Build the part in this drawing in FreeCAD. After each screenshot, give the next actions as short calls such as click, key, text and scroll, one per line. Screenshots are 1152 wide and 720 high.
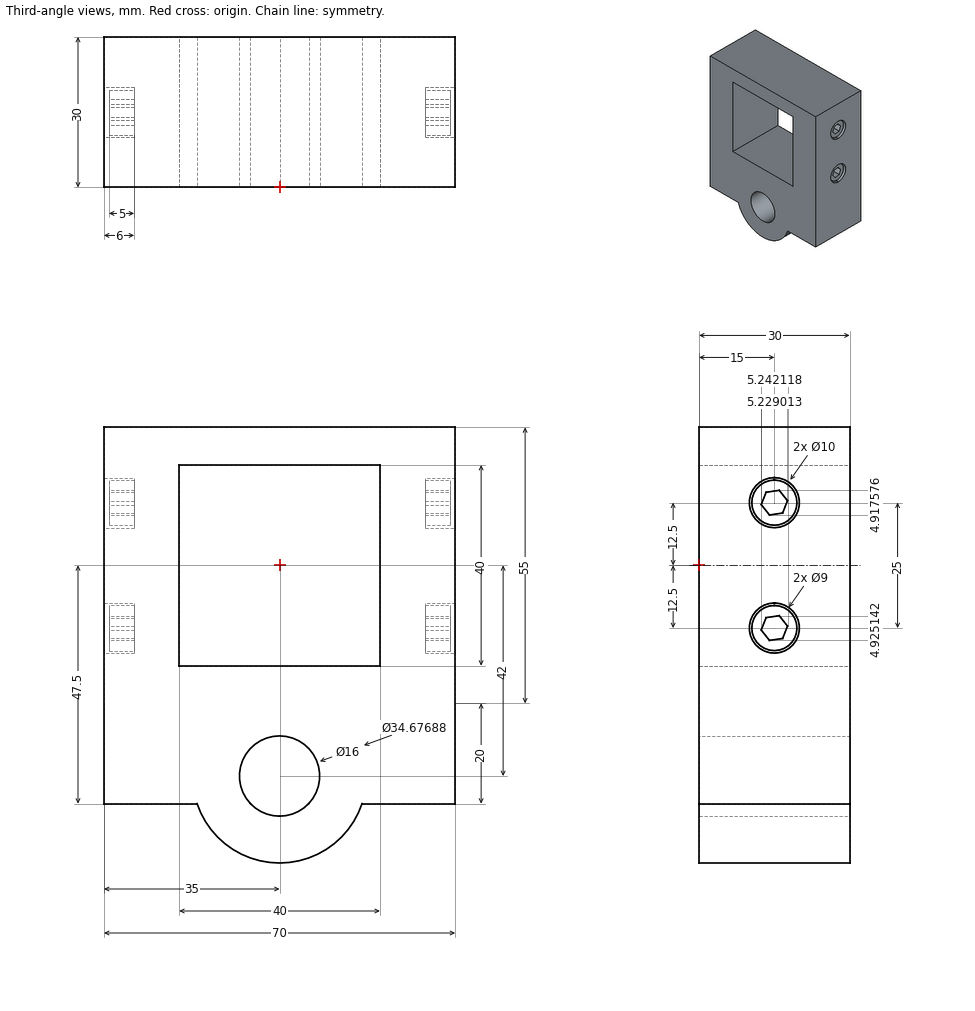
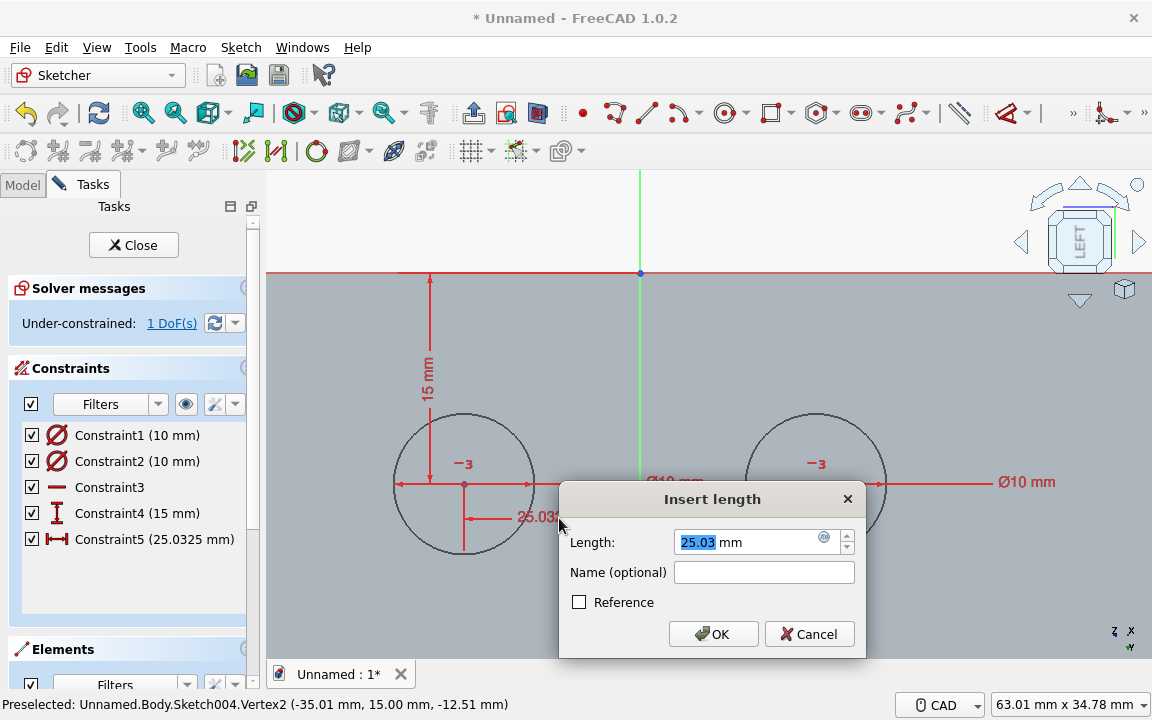
text(25)
key(Return)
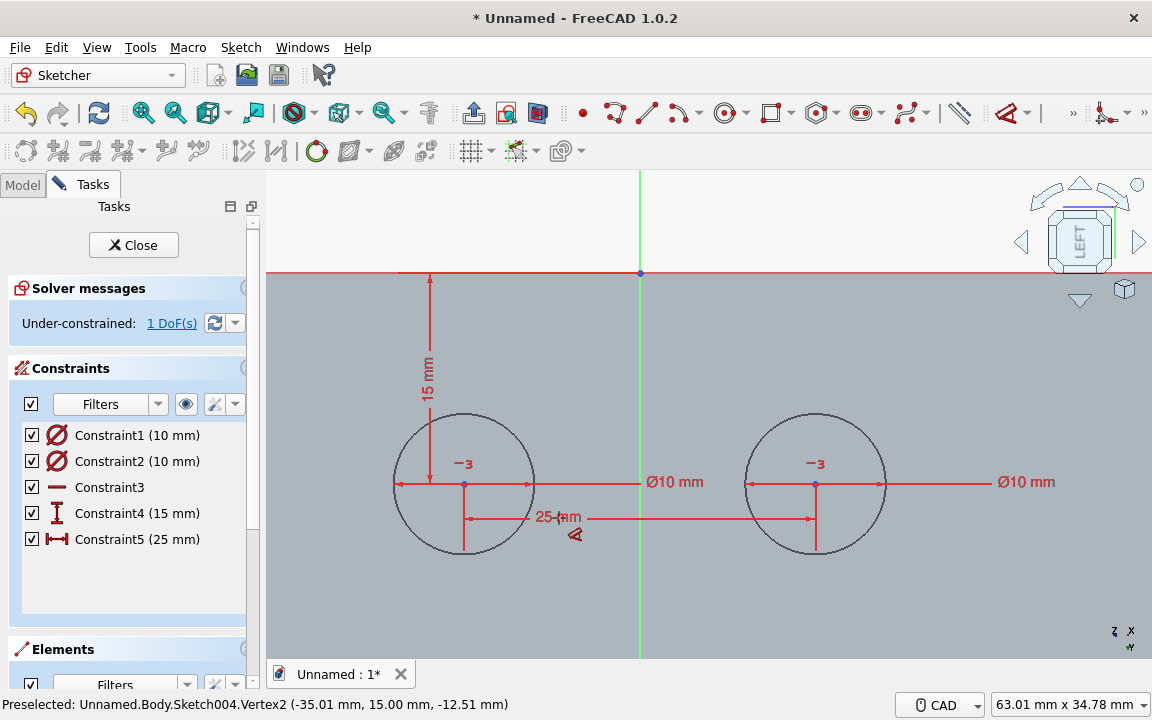
click(464, 484)
click(552, 239)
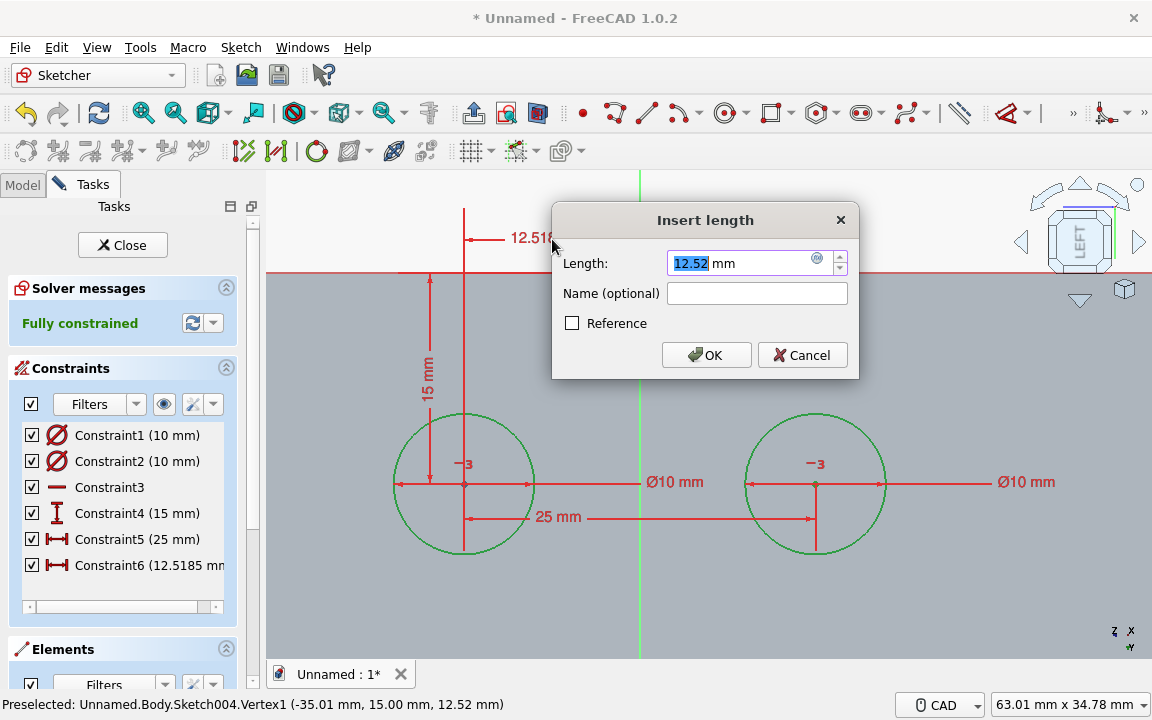
text(12.5)
key(Return)
key(Escape)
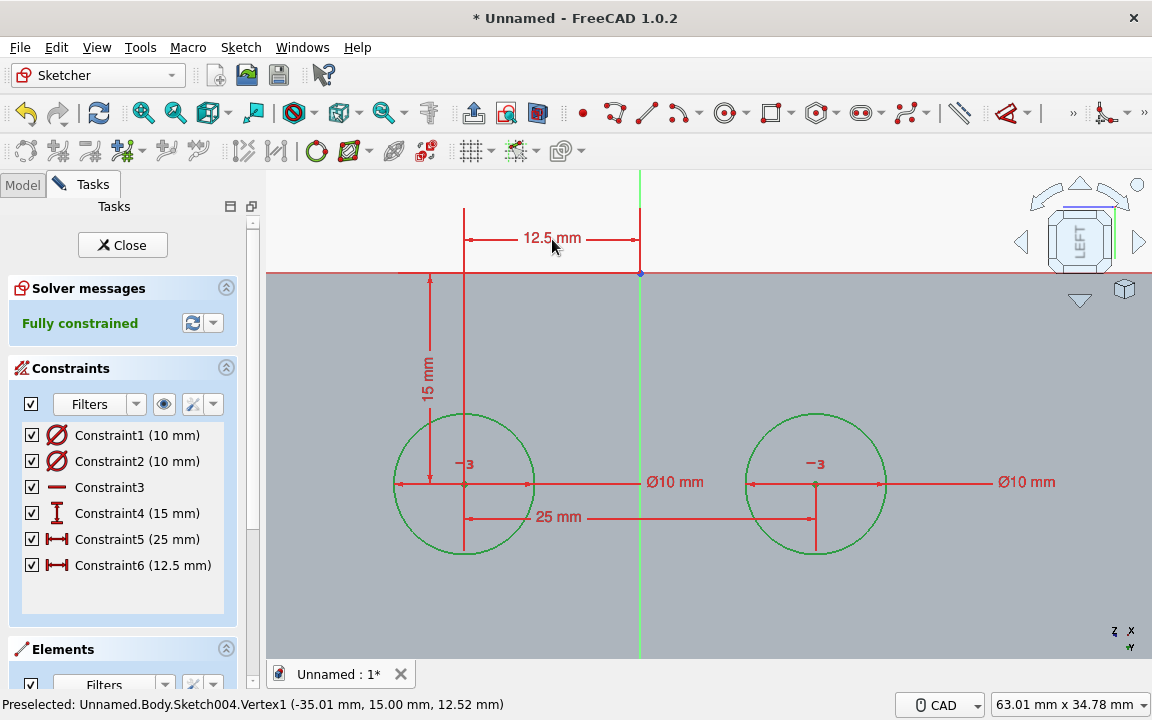
click(123, 245)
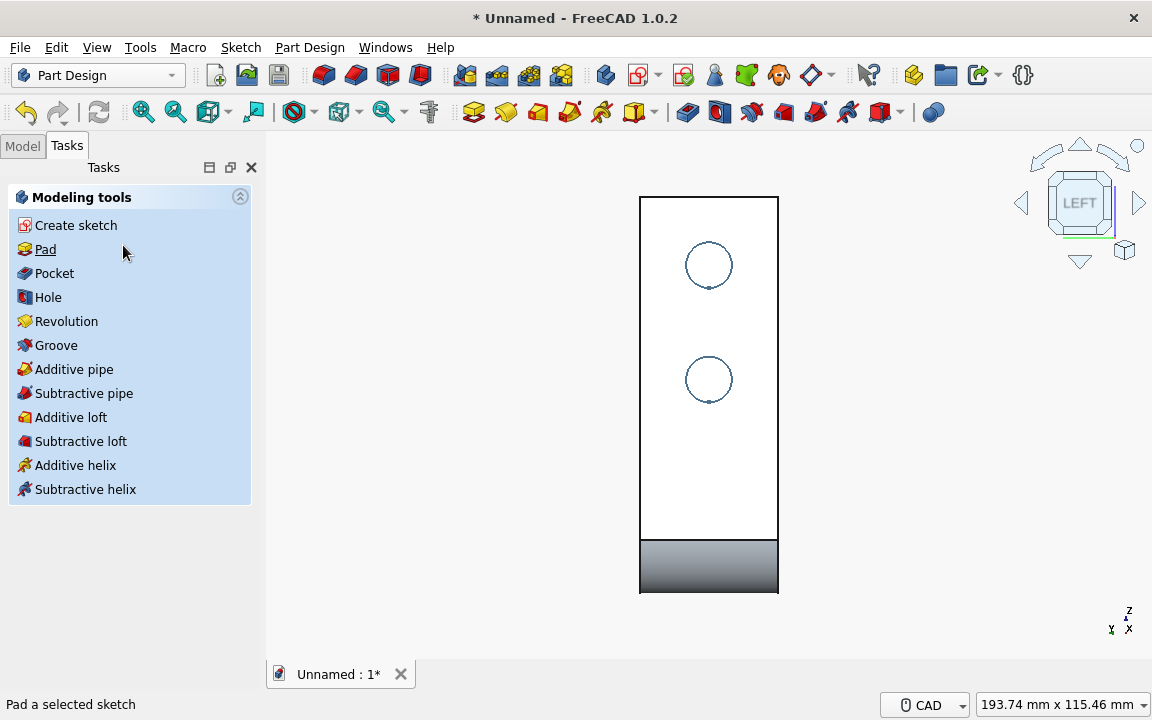
click(688, 112)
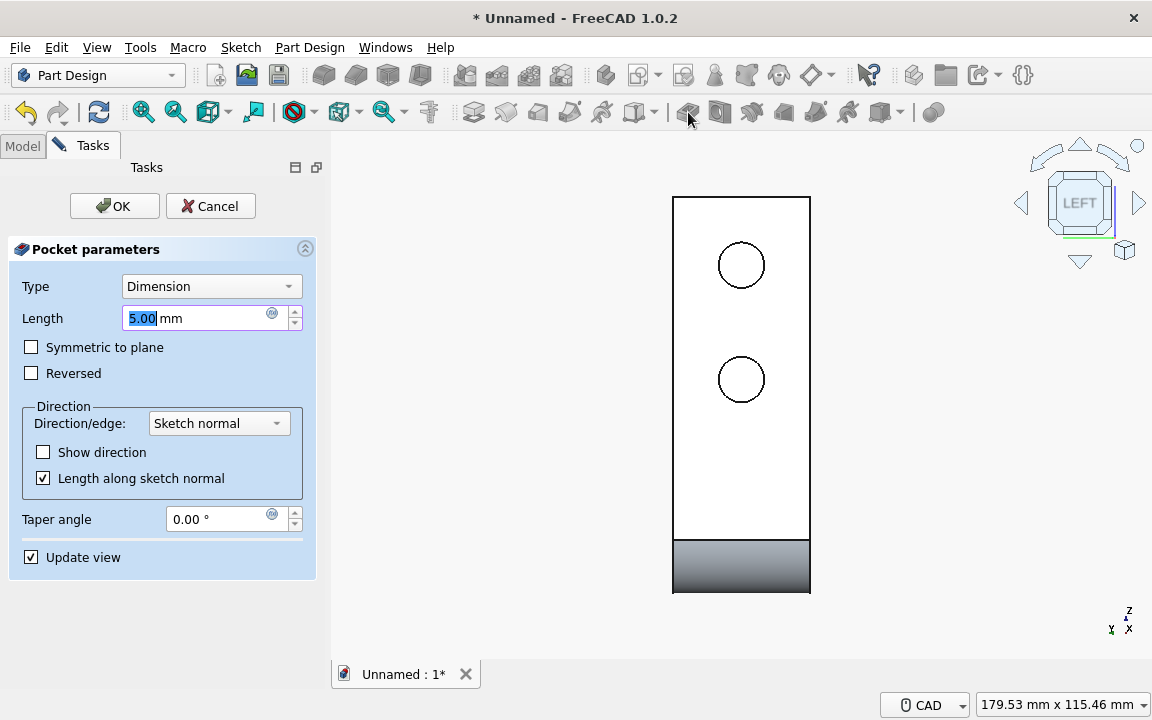
text(6)
key(Tab)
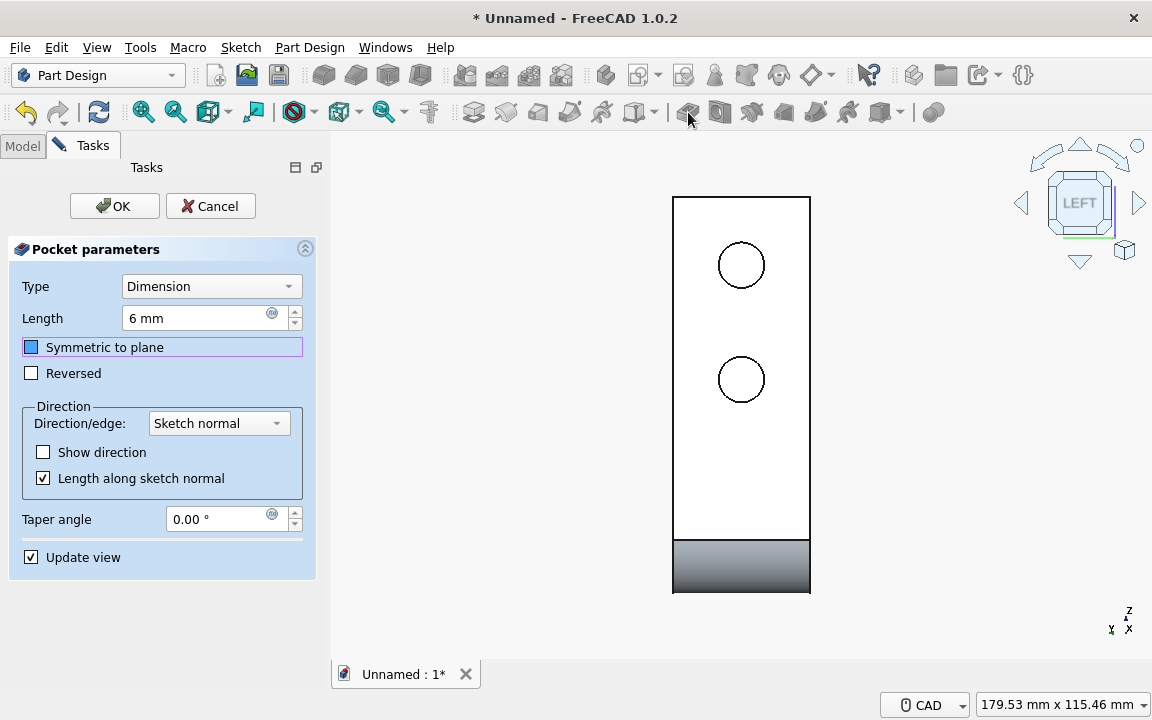
click(115, 206)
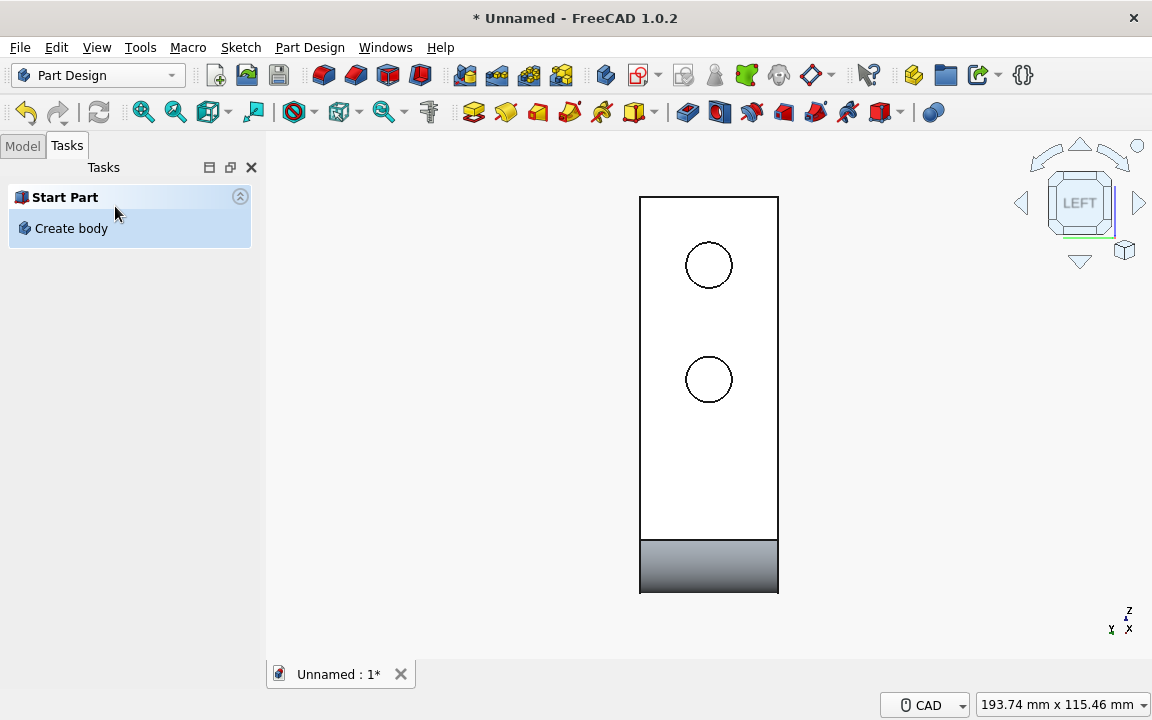
click(709, 264)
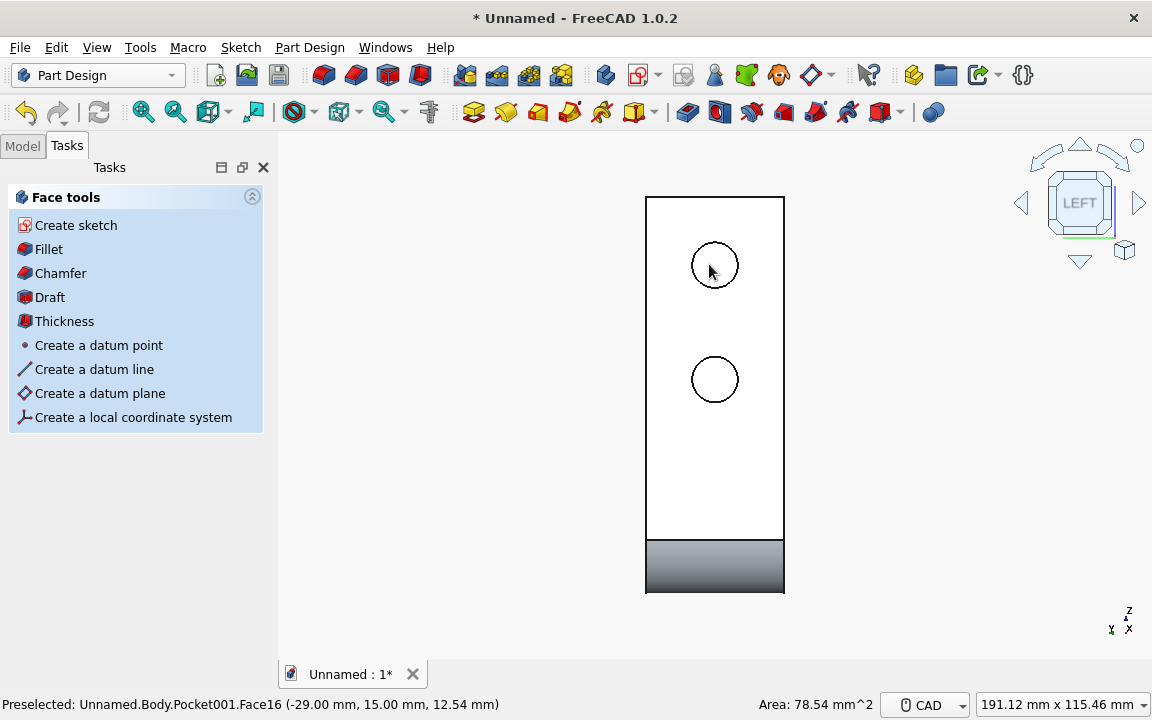
click(638, 76)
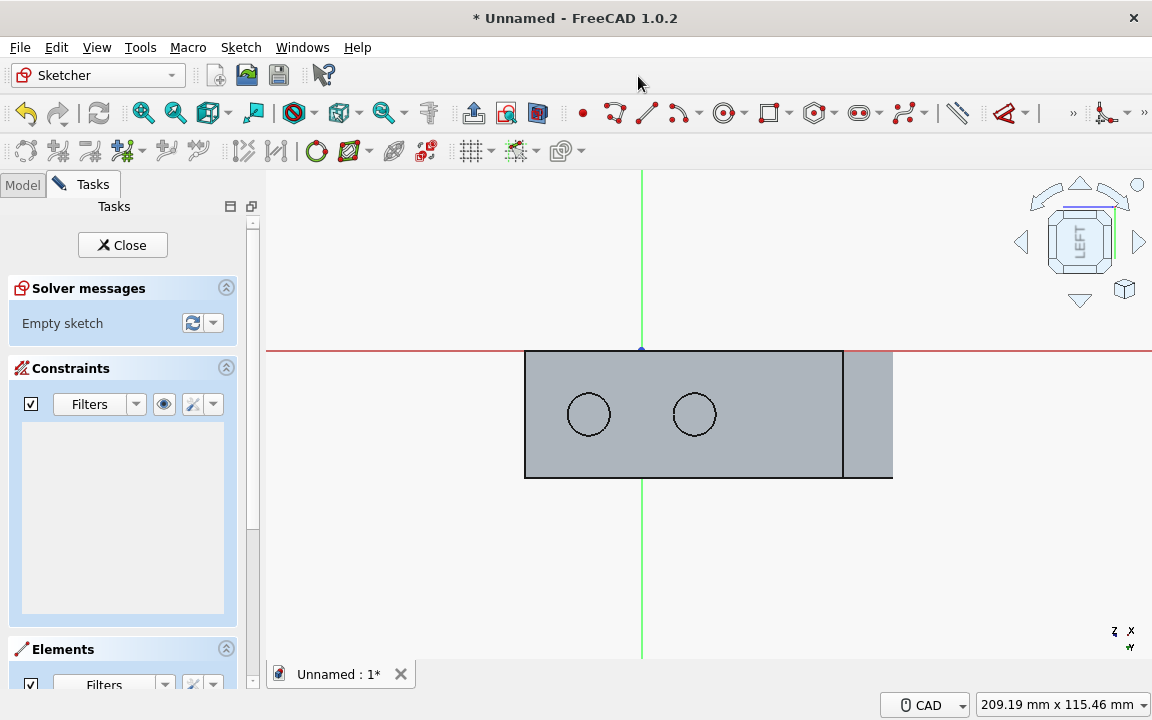
click(538, 114)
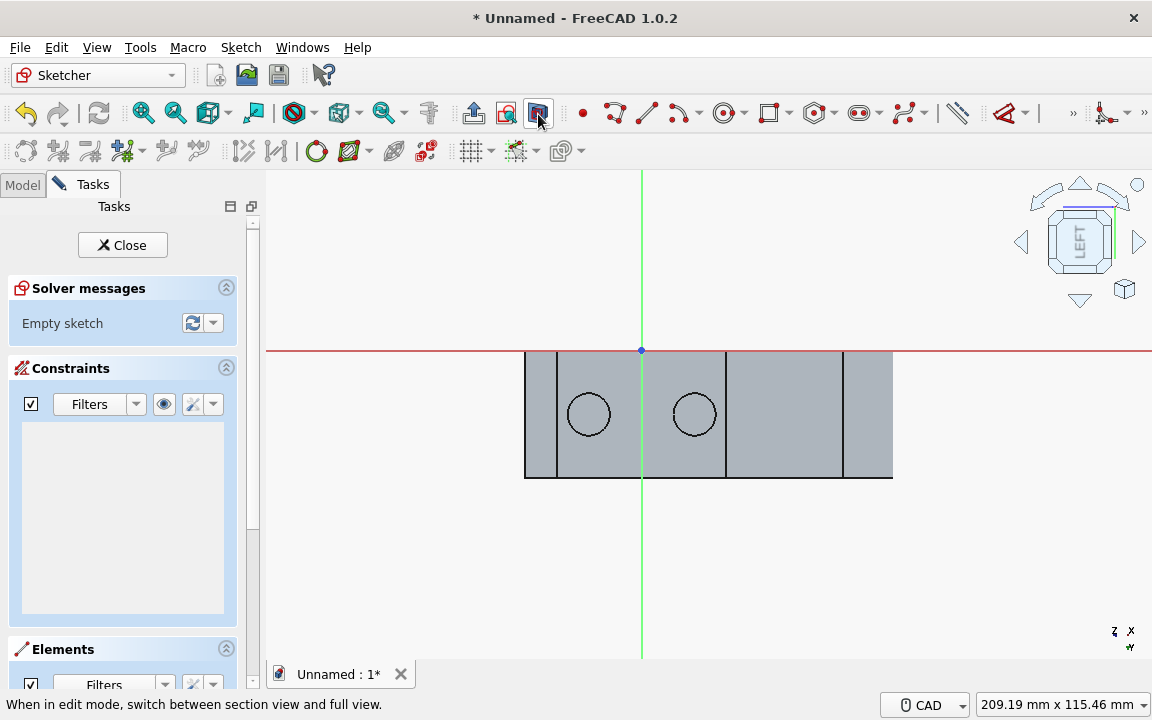
scroll(642, 383, up, 6)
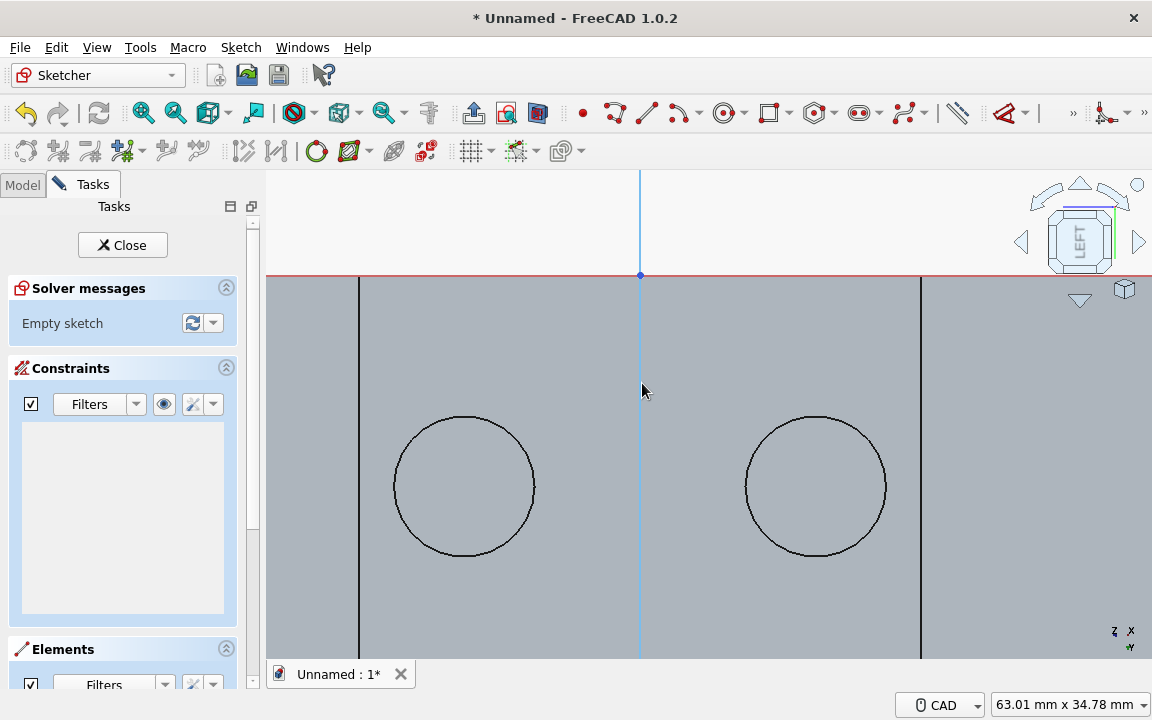
click(814, 114)